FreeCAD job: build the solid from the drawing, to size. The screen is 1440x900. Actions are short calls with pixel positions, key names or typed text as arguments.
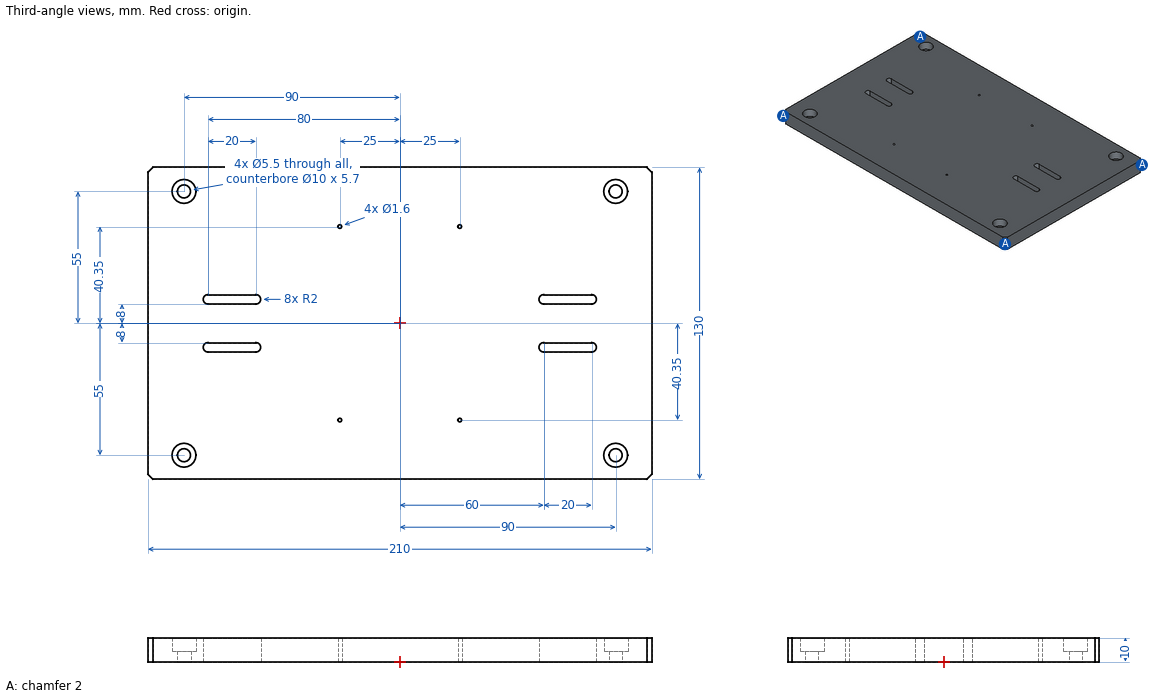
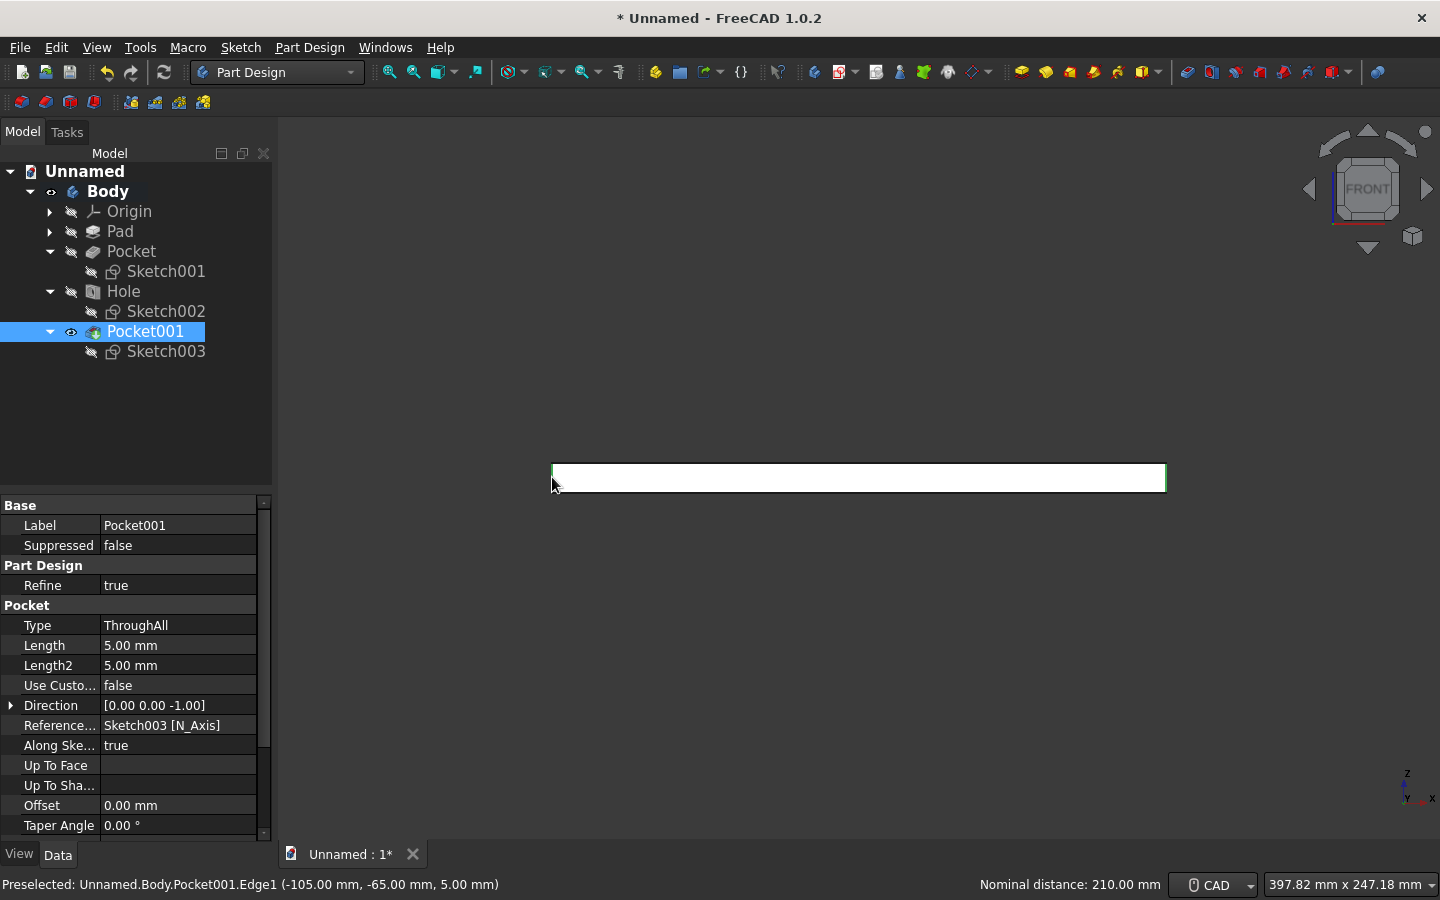
key(3)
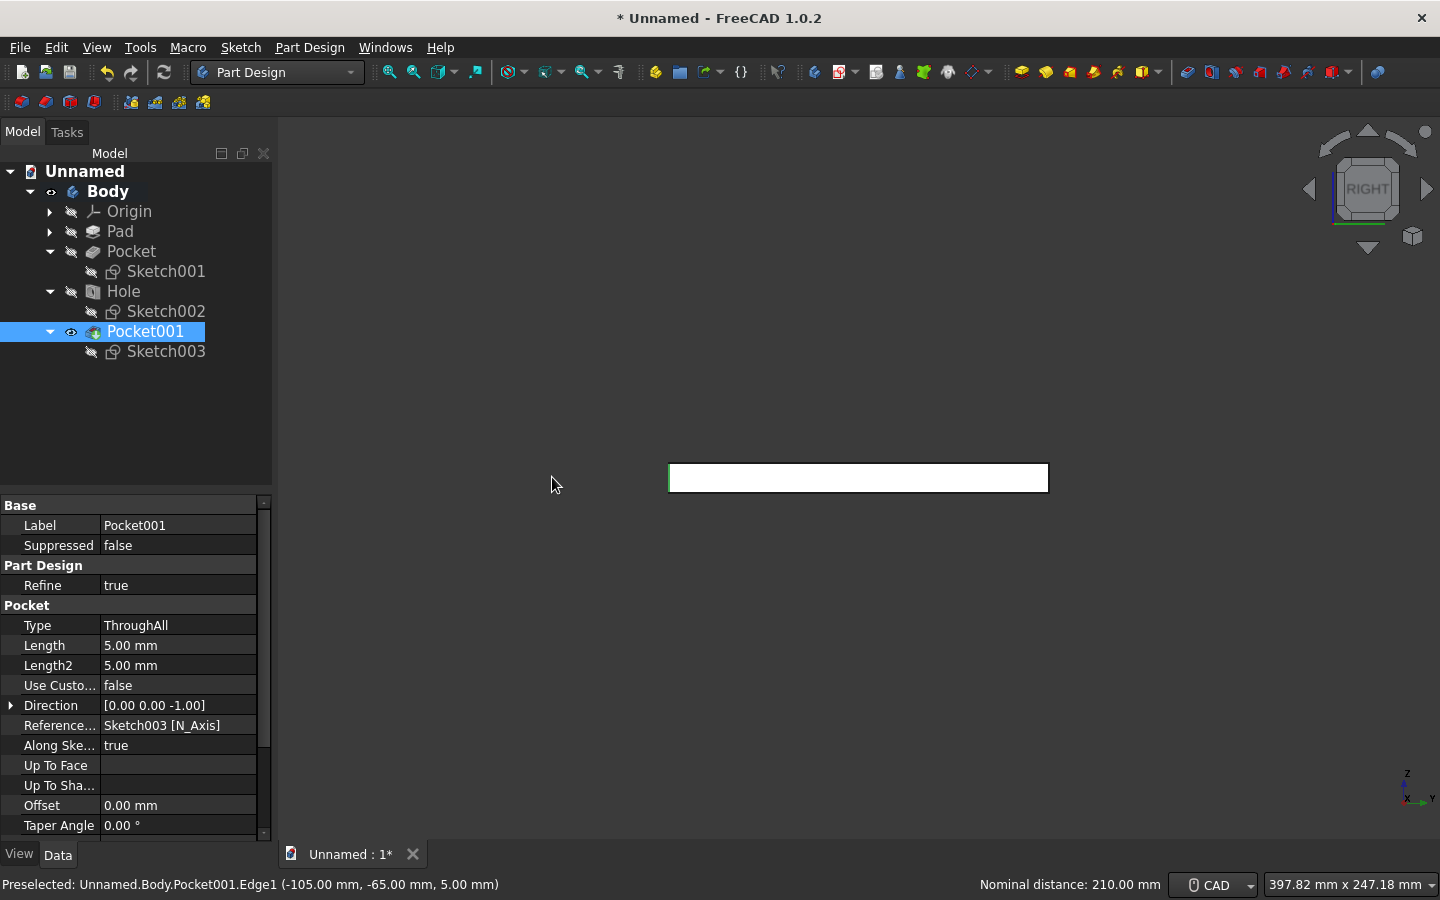
click(390, 72)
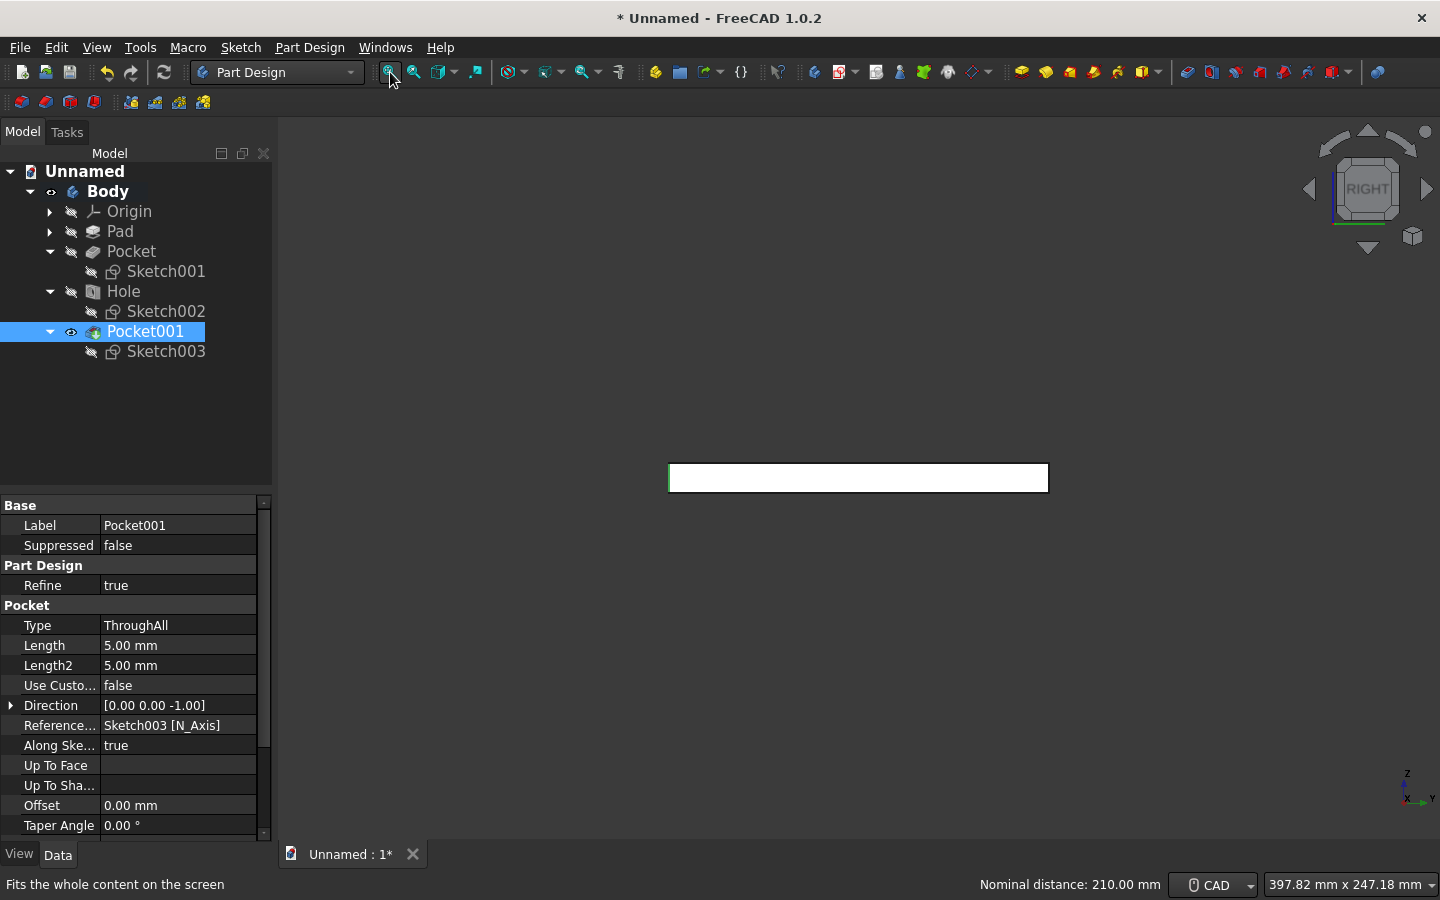
click(1049, 477, ctrl)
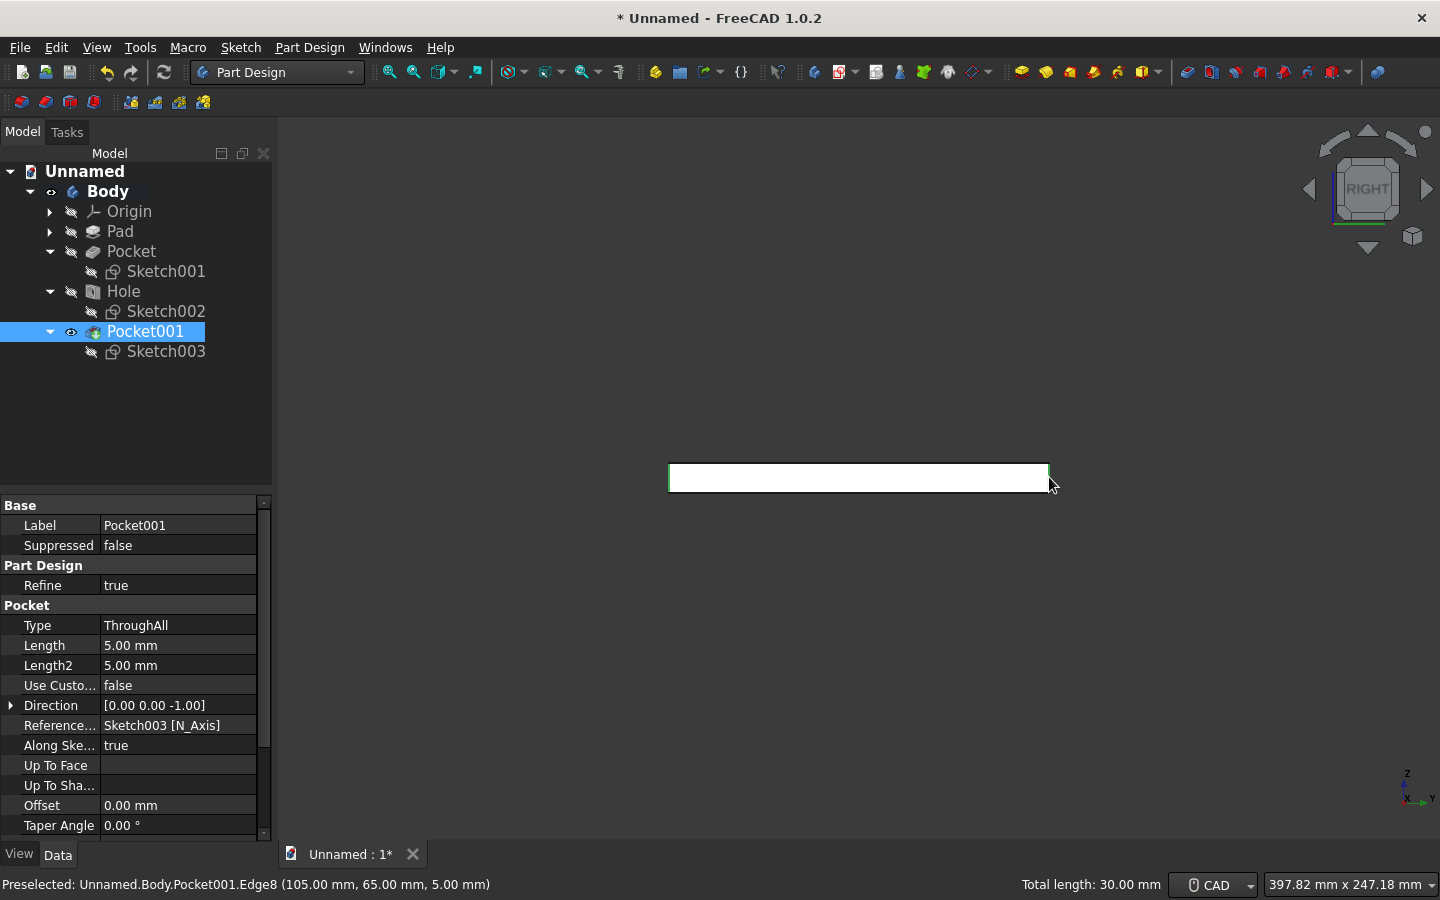
key(5)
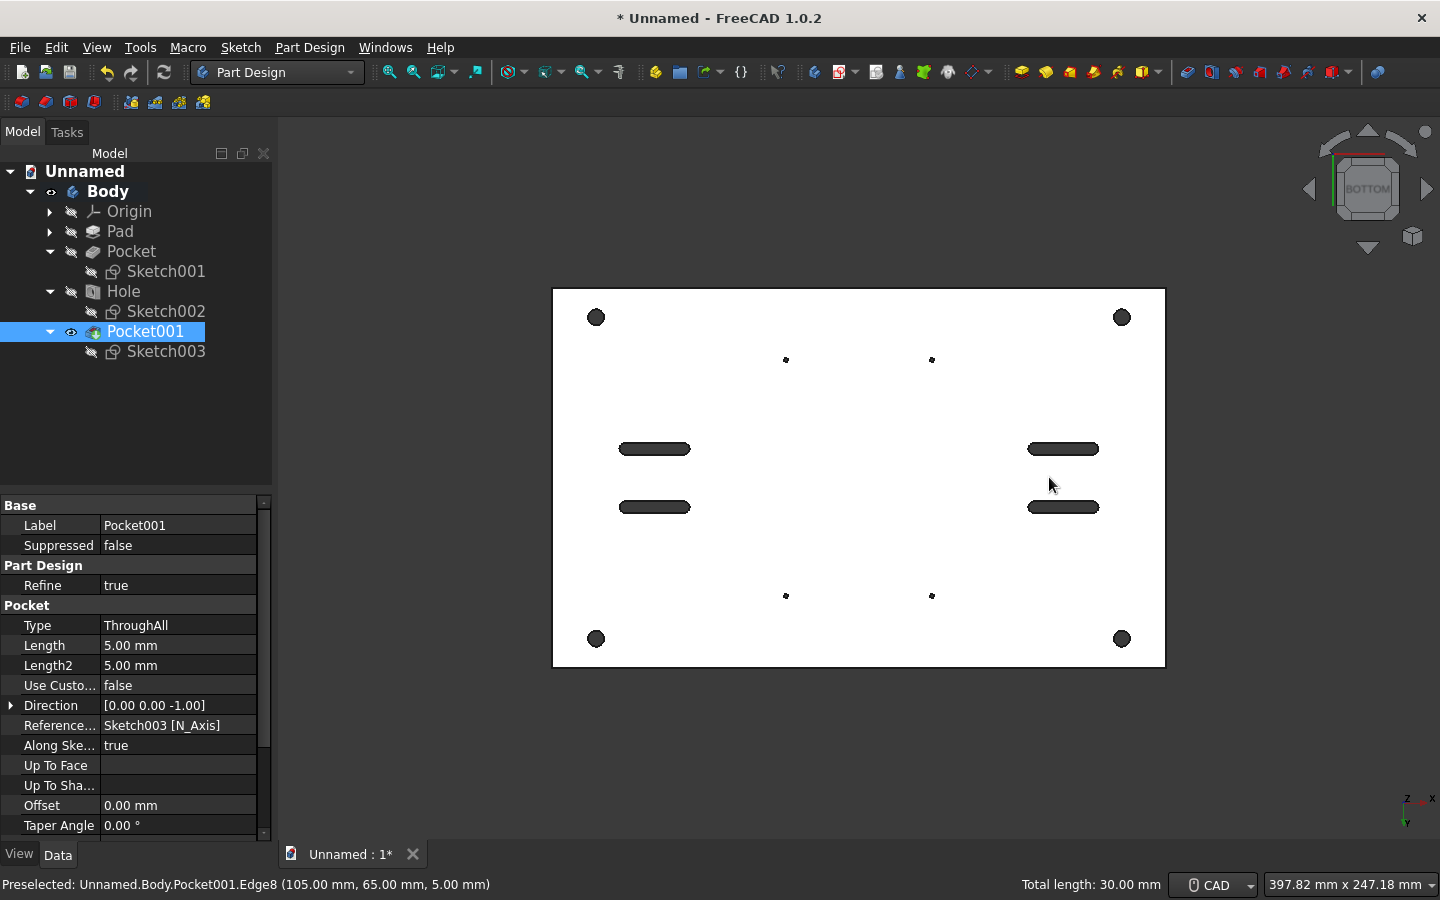
key(4)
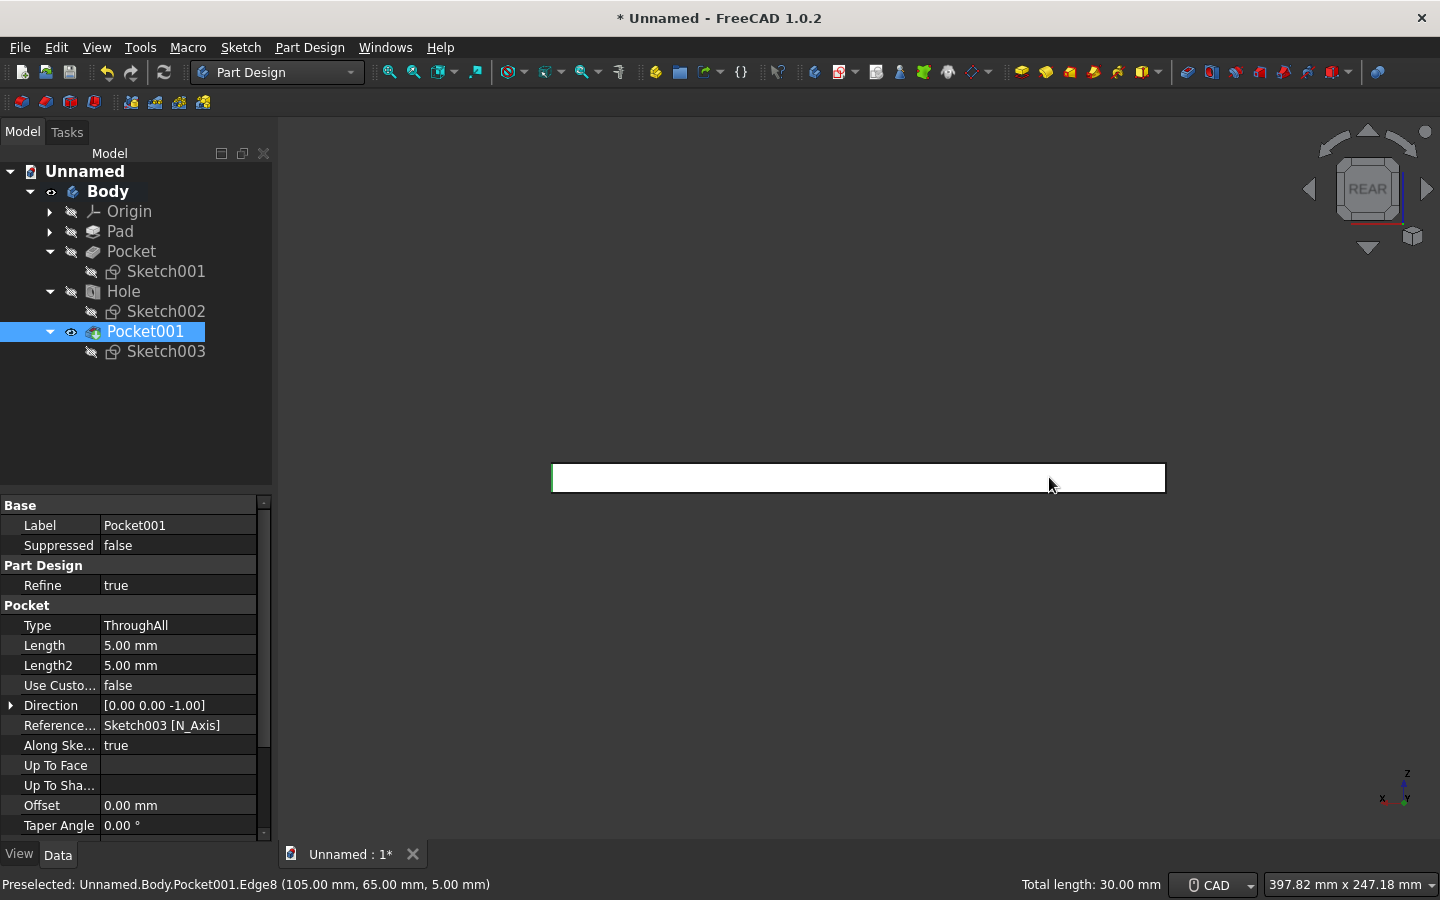
click(1166, 477, ctrl)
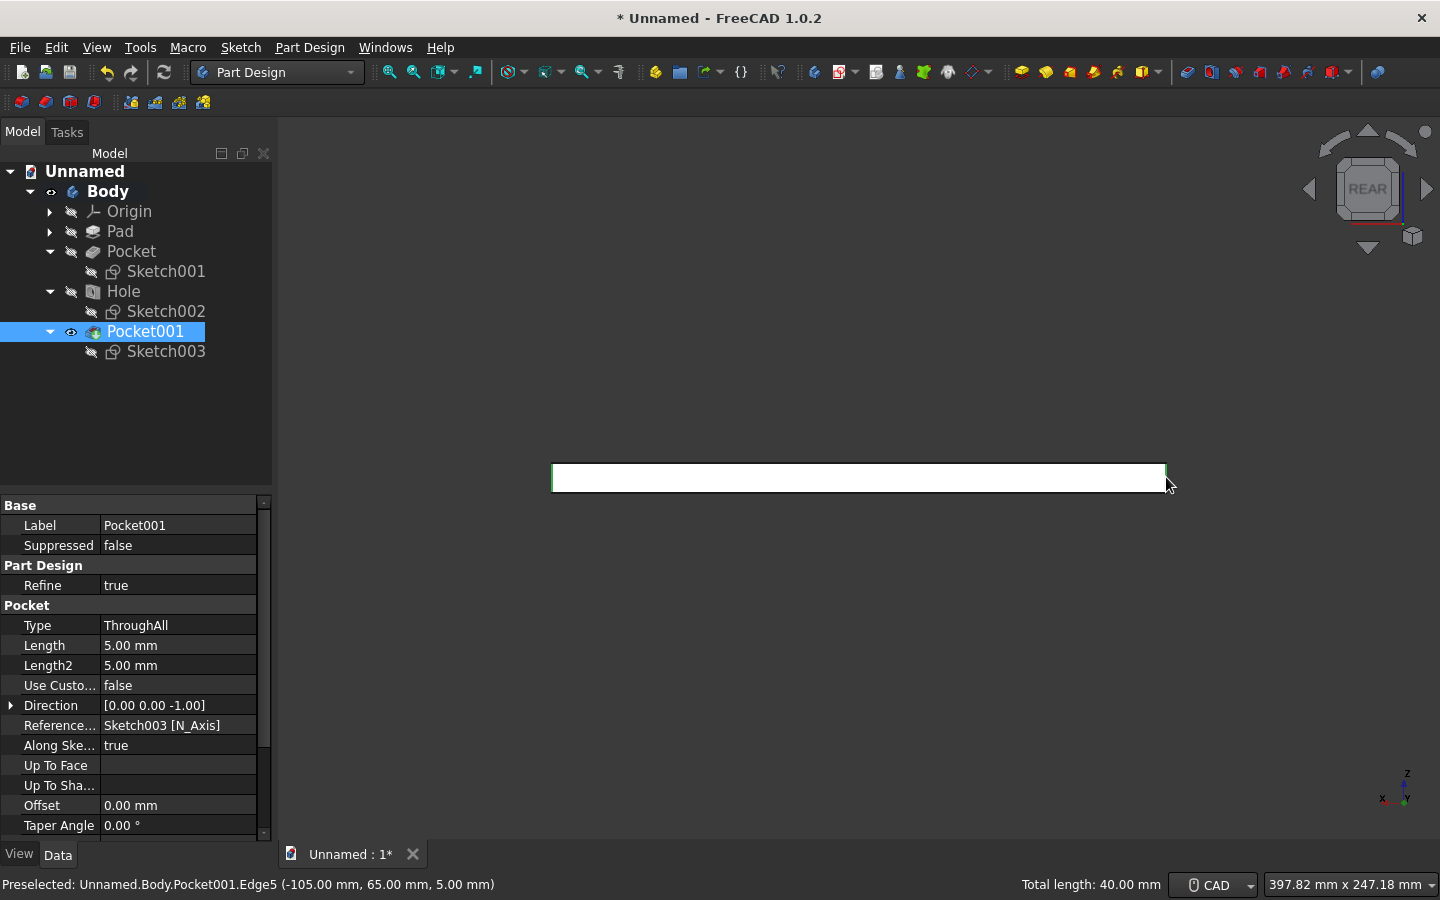
click(46, 102)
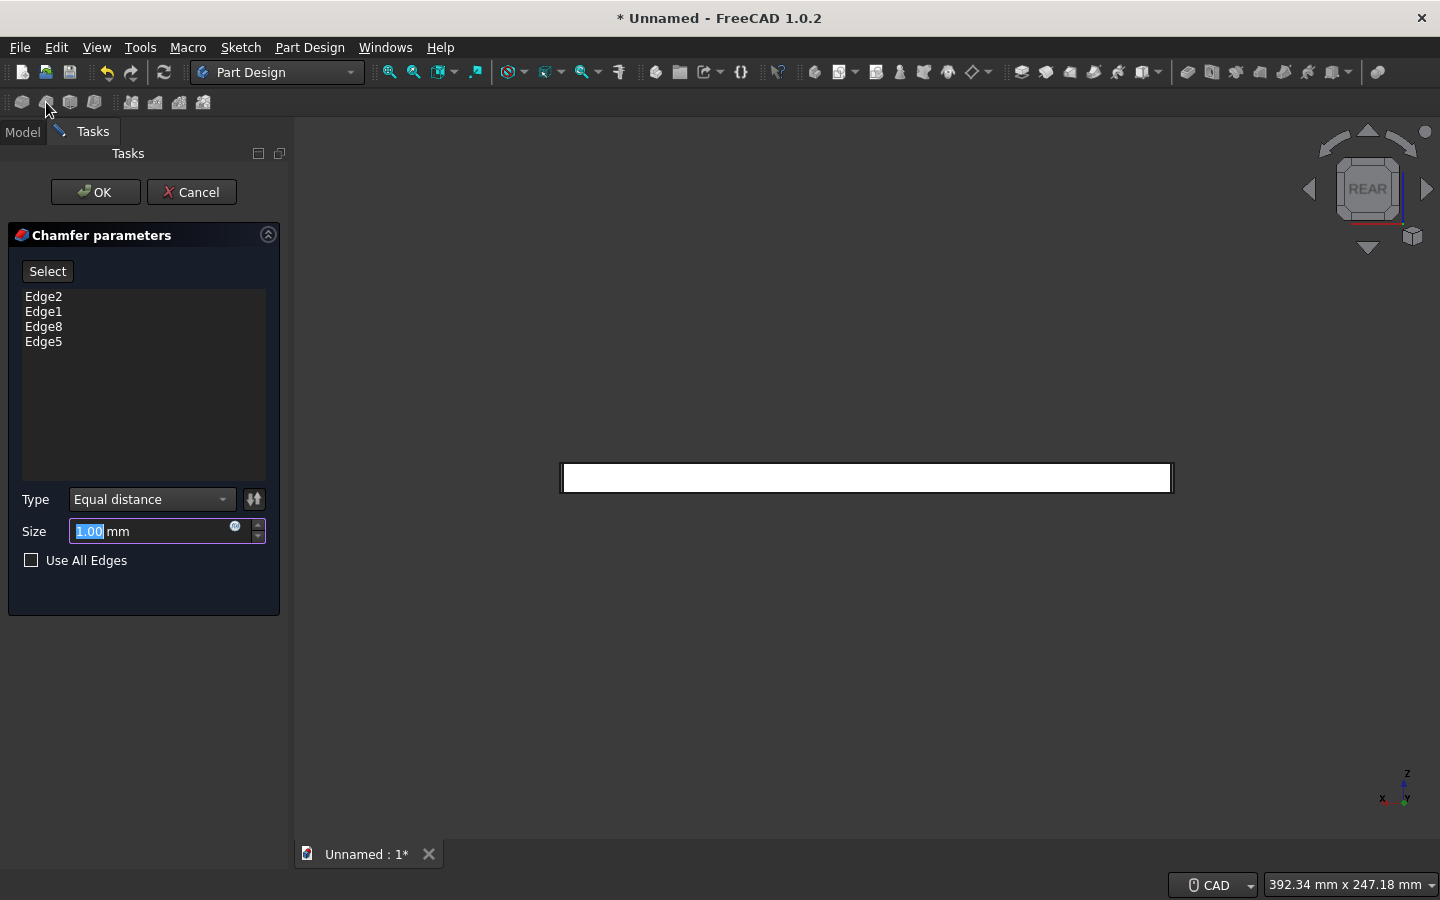
text(2)
key(Tab)